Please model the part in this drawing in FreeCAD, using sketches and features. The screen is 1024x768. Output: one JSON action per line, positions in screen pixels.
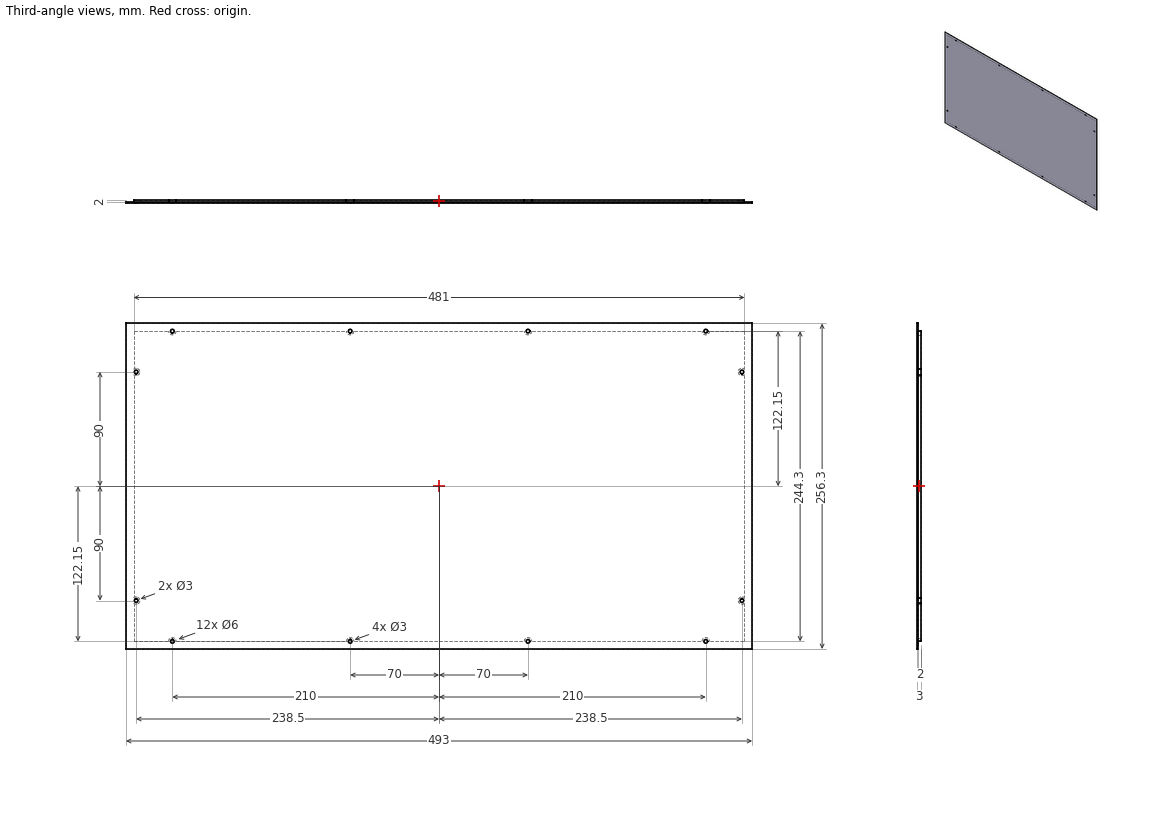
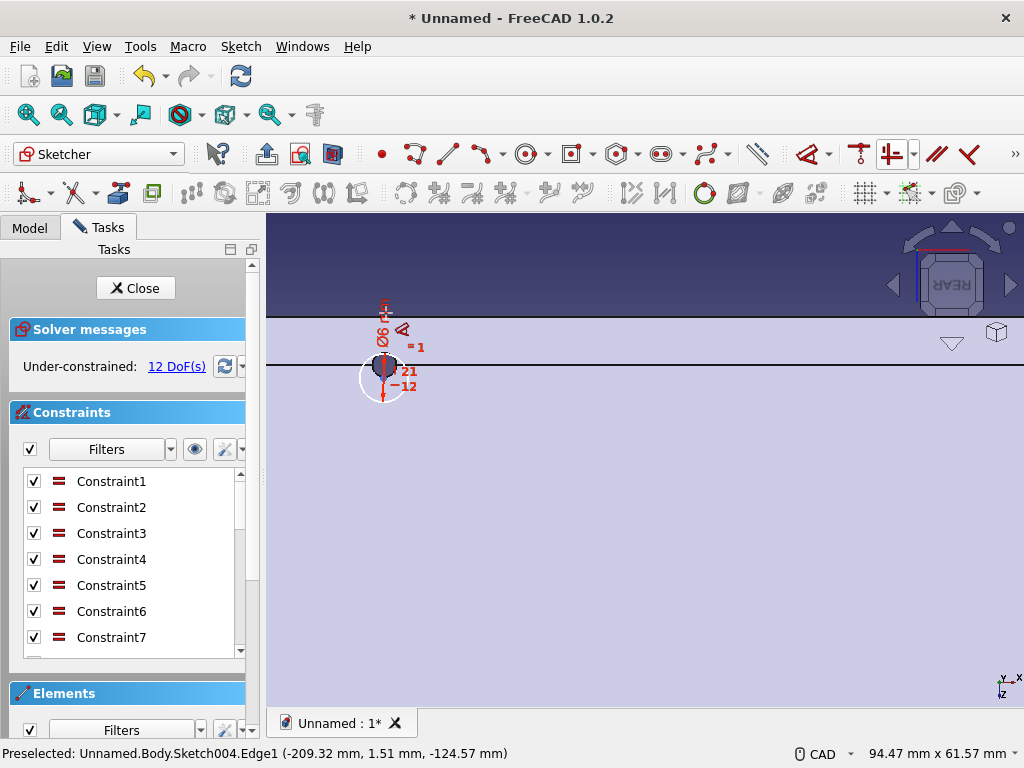
{"action": "scroll", "coordinate": [390, 350], "scroll_direction": "down", "scroll_amount": 11}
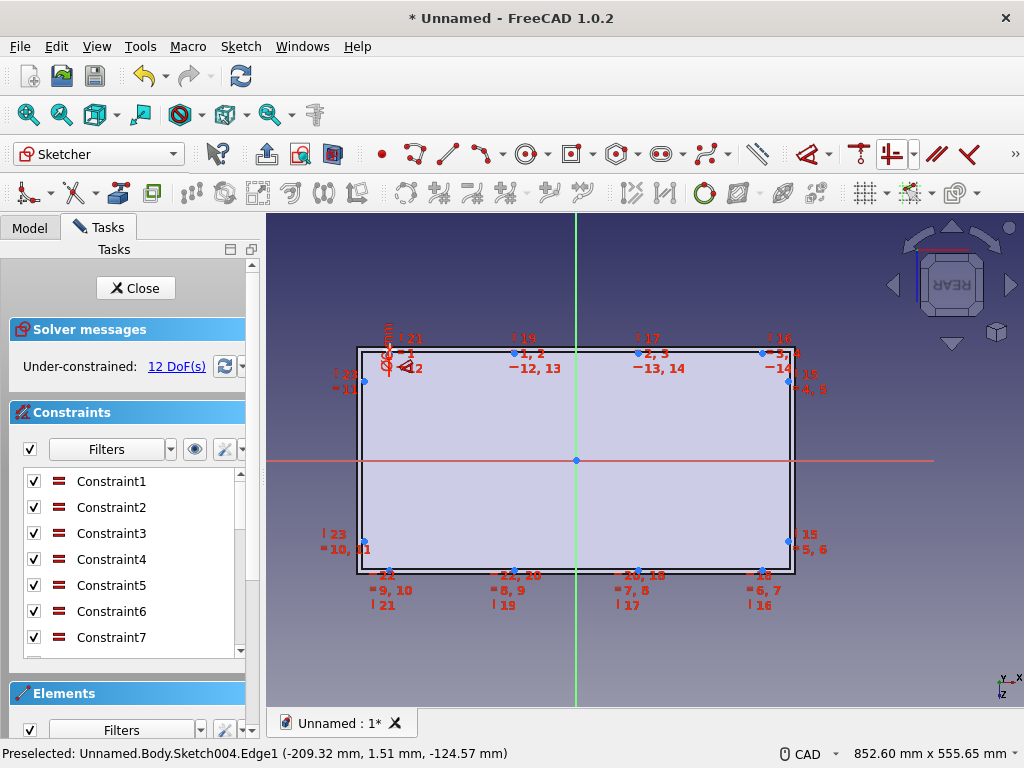
{"action": "left_click", "coordinate": [514, 353]}
{"action": "left_click", "coordinate": [545, 319]}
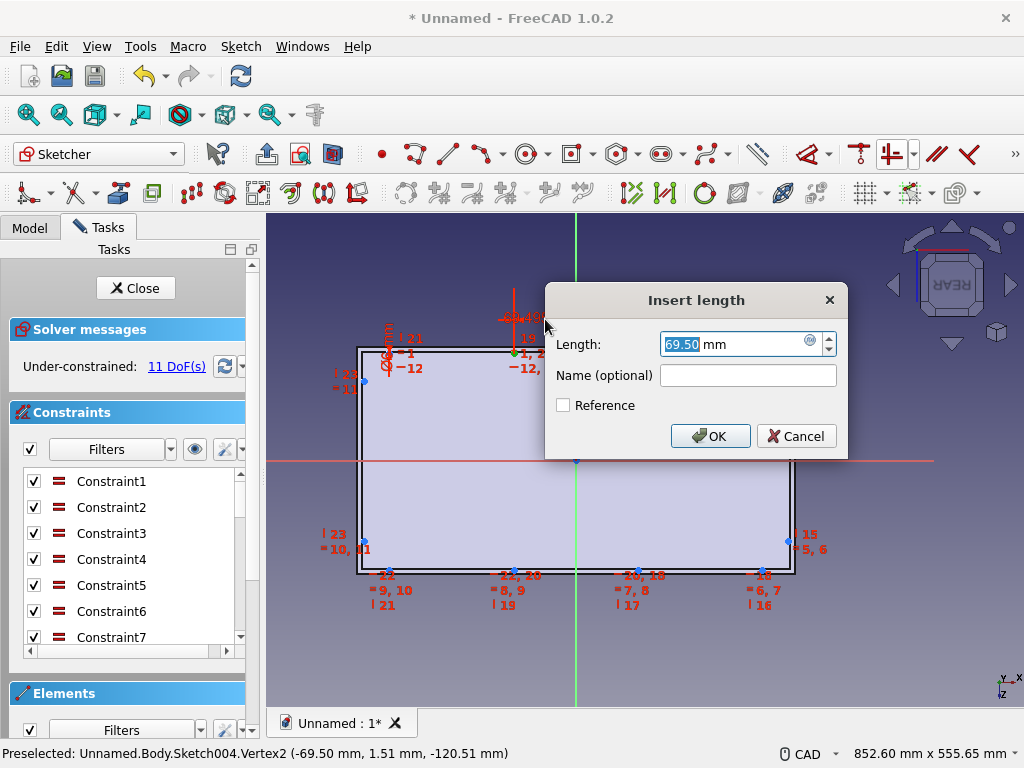
{"action": "type", "text": "70"}
{"action": "key", "text": "Return"}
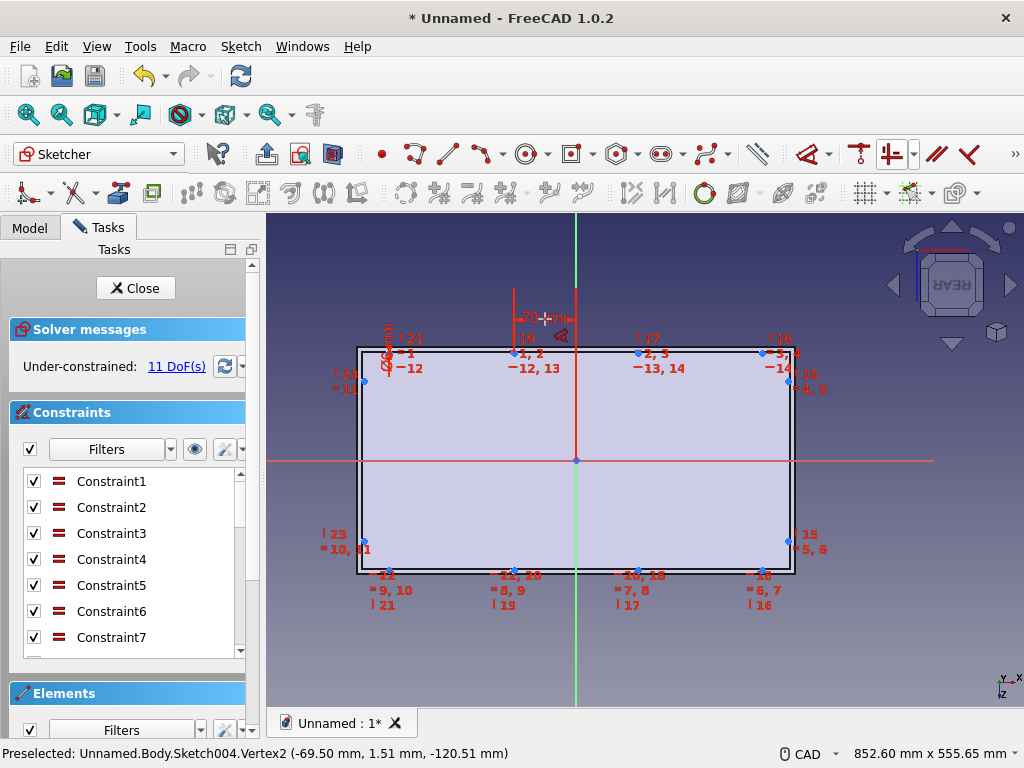
{"action": "left_click", "coordinate": [638, 353]}
{"action": "left_click", "coordinate": [622, 319]}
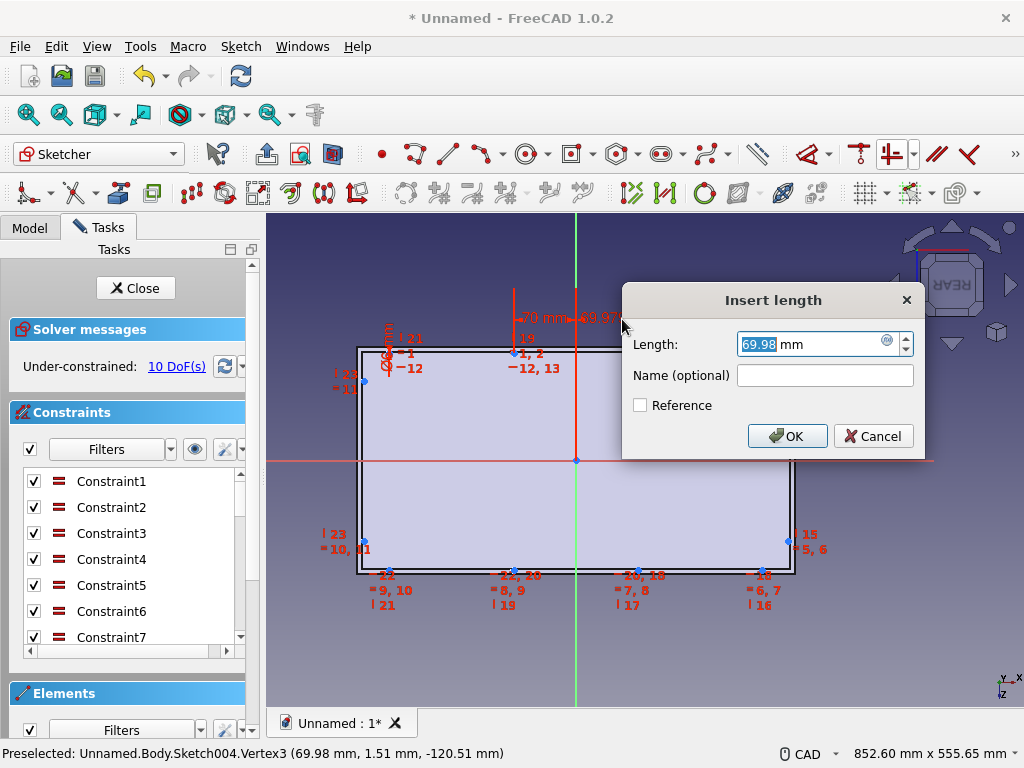
{"action": "type", "text": "70"}
{"action": "key", "text": "Return"}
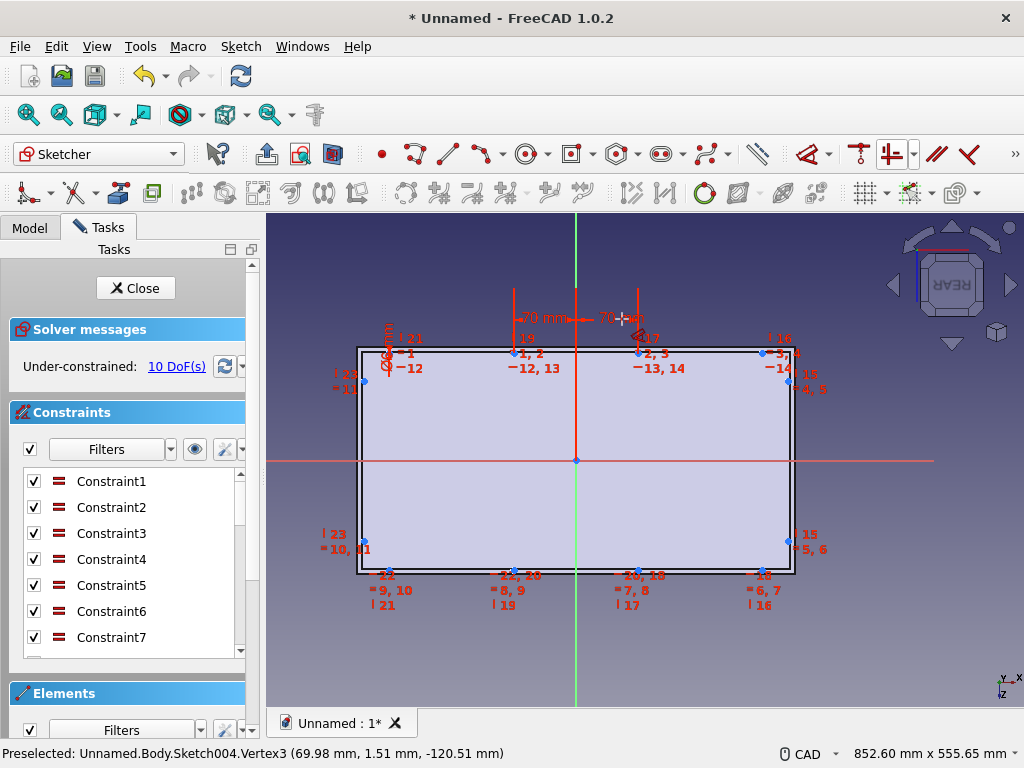
{"action": "left_click", "coordinate": [788, 381]}
{"action": "left_click", "coordinate": [822, 421]}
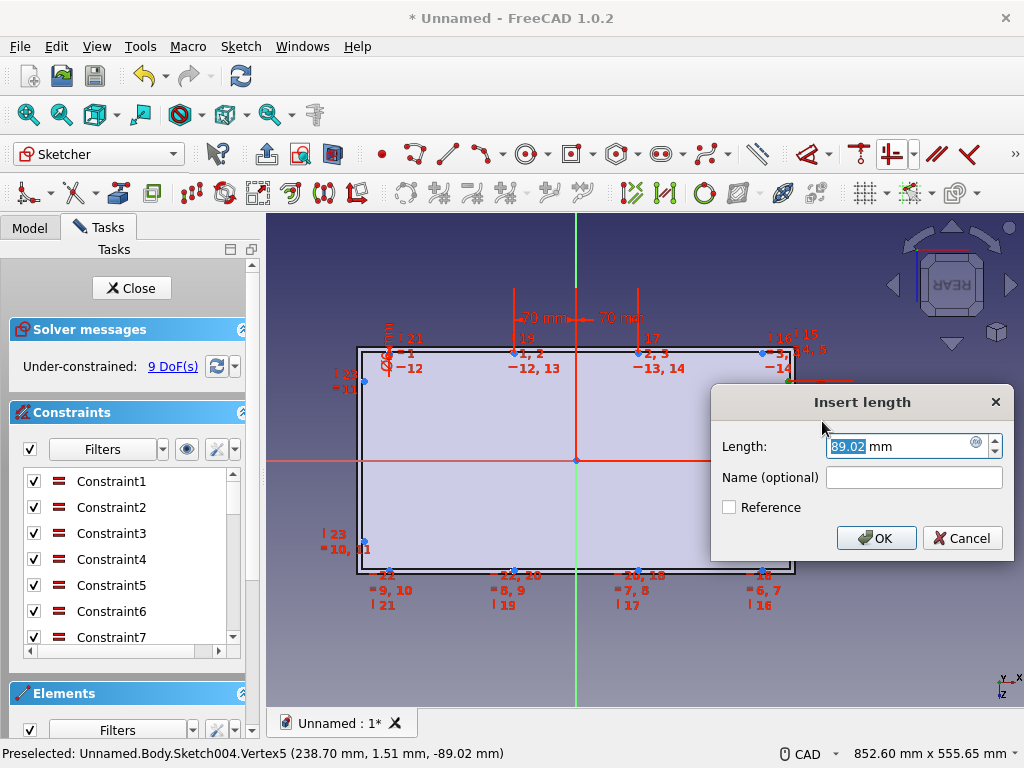
{"action": "type", "text": "90"}
{"action": "key", "text": "Return"}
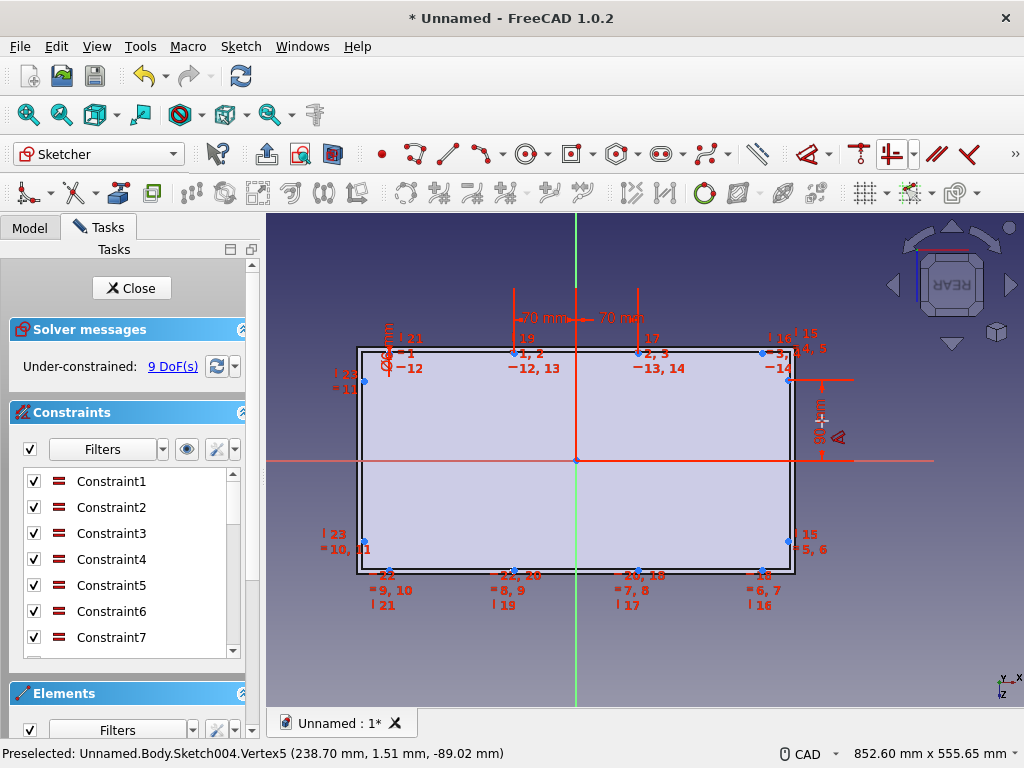
{"action": "left_click", "coordinate": [788, 541]}
{"action": "left_click", "coordinate": [822, 501]}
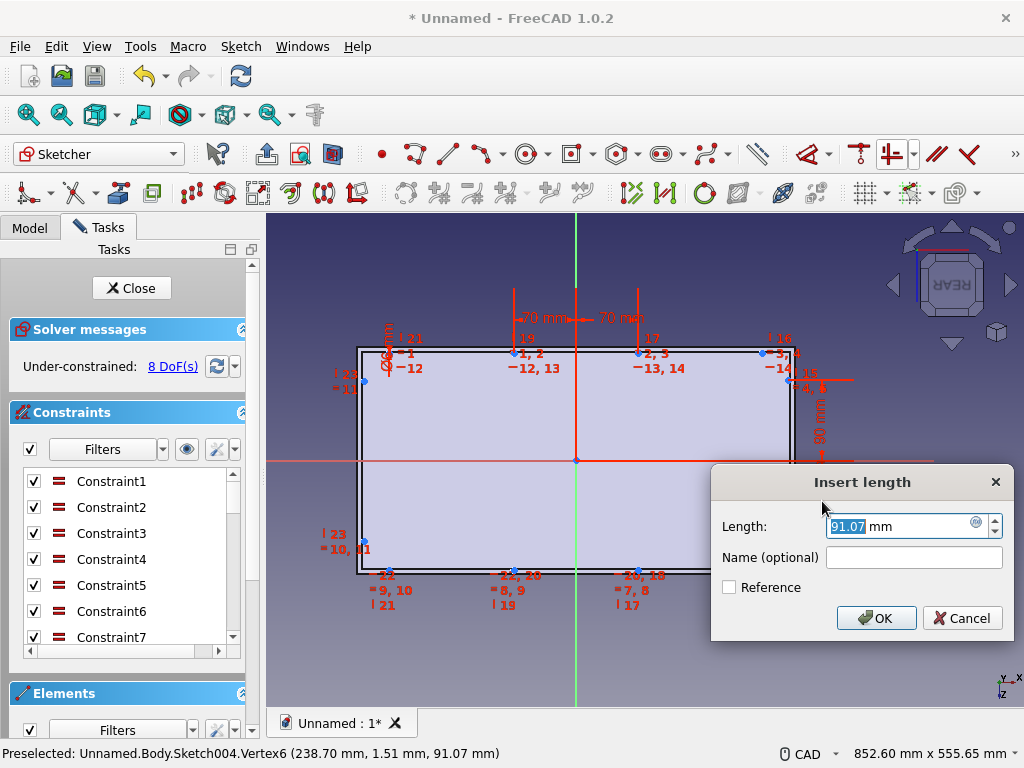
{"action": "type", "text": "90"}
{"action": "key", "text": "Return"}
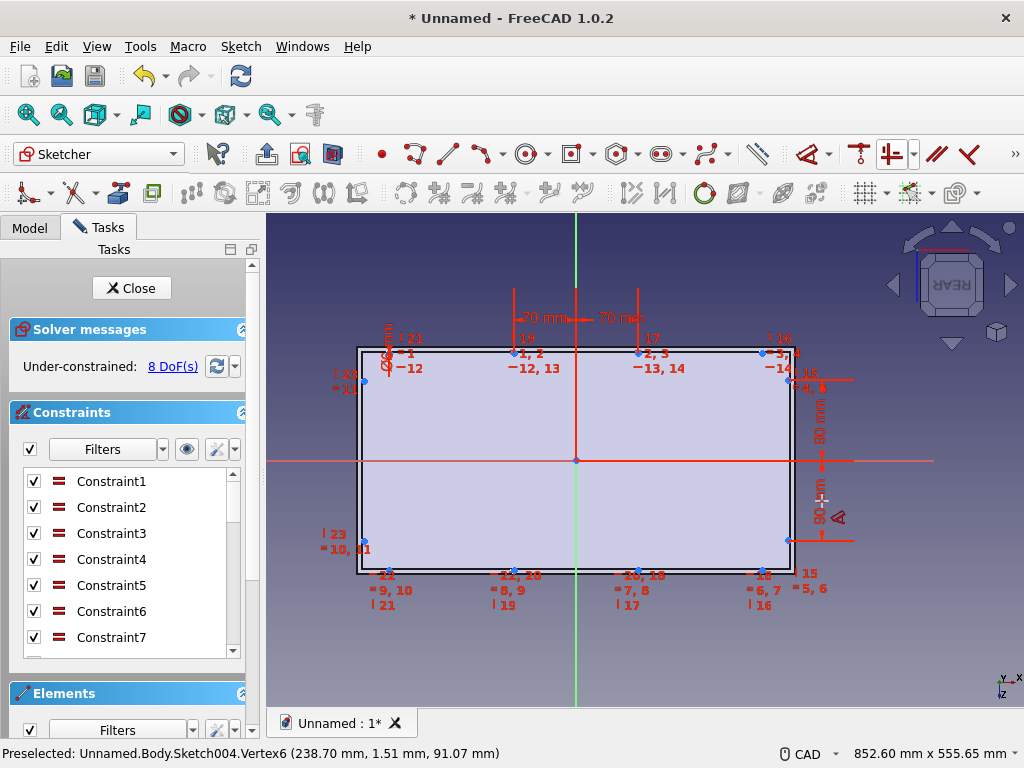
{"action": "left_click", "coordinate": [364, 541]}
{"action": "left_click", "coordinate": [330, 501]}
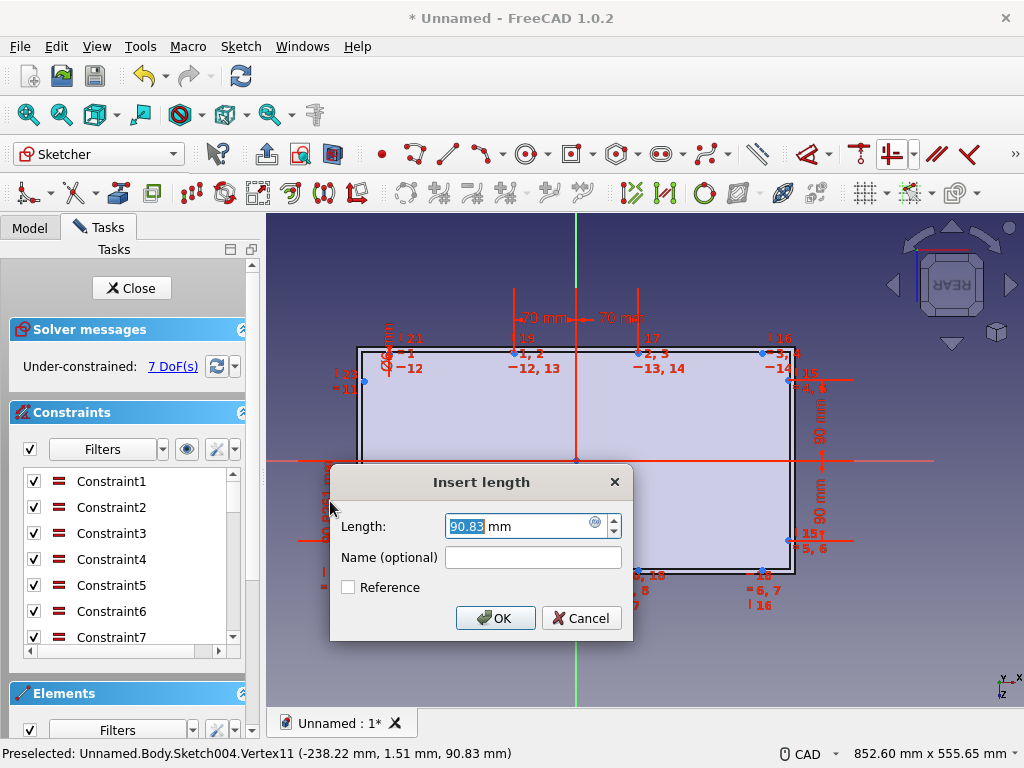
{"action": "type", "text": "90"}
{"action": "key", "text": "Return"}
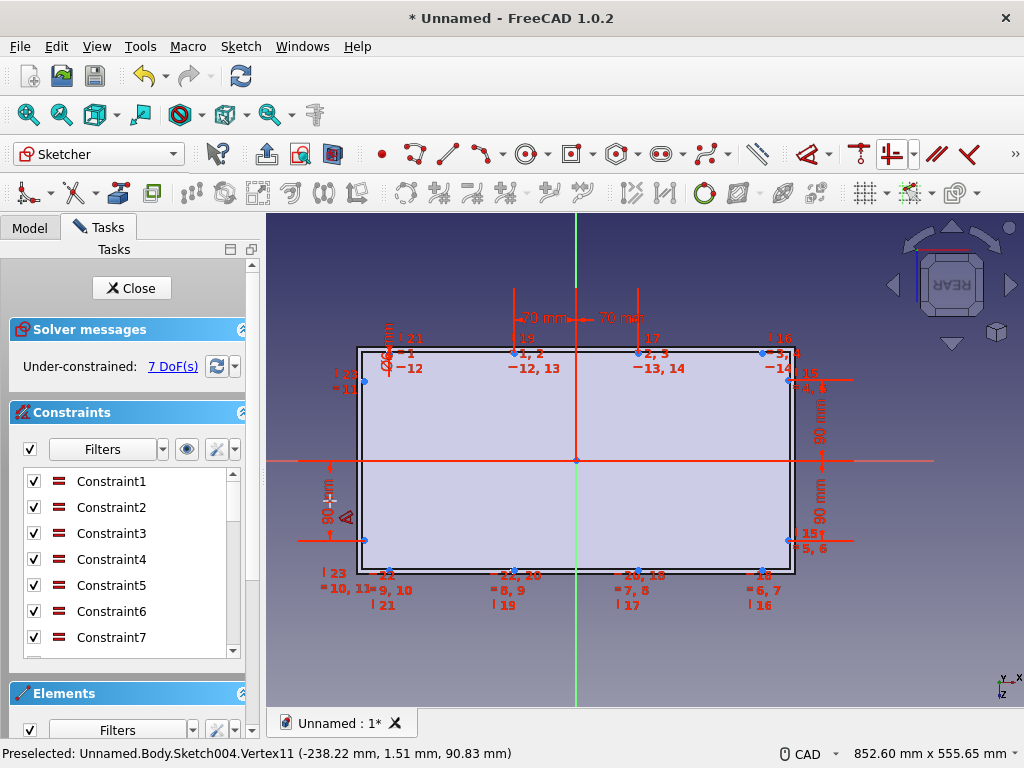
{"action": "left_click", "coordinate": [364, 381]}
{"action": "left_click", "coordinate": [330, 421]}